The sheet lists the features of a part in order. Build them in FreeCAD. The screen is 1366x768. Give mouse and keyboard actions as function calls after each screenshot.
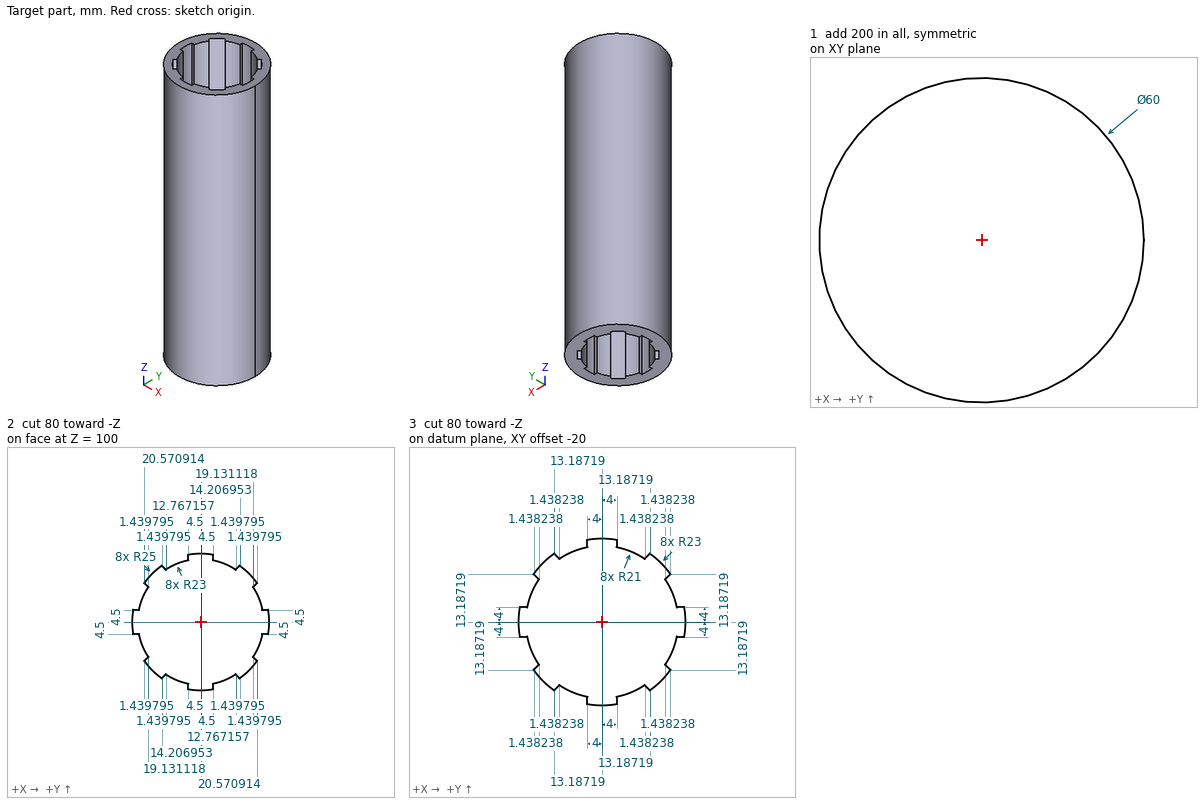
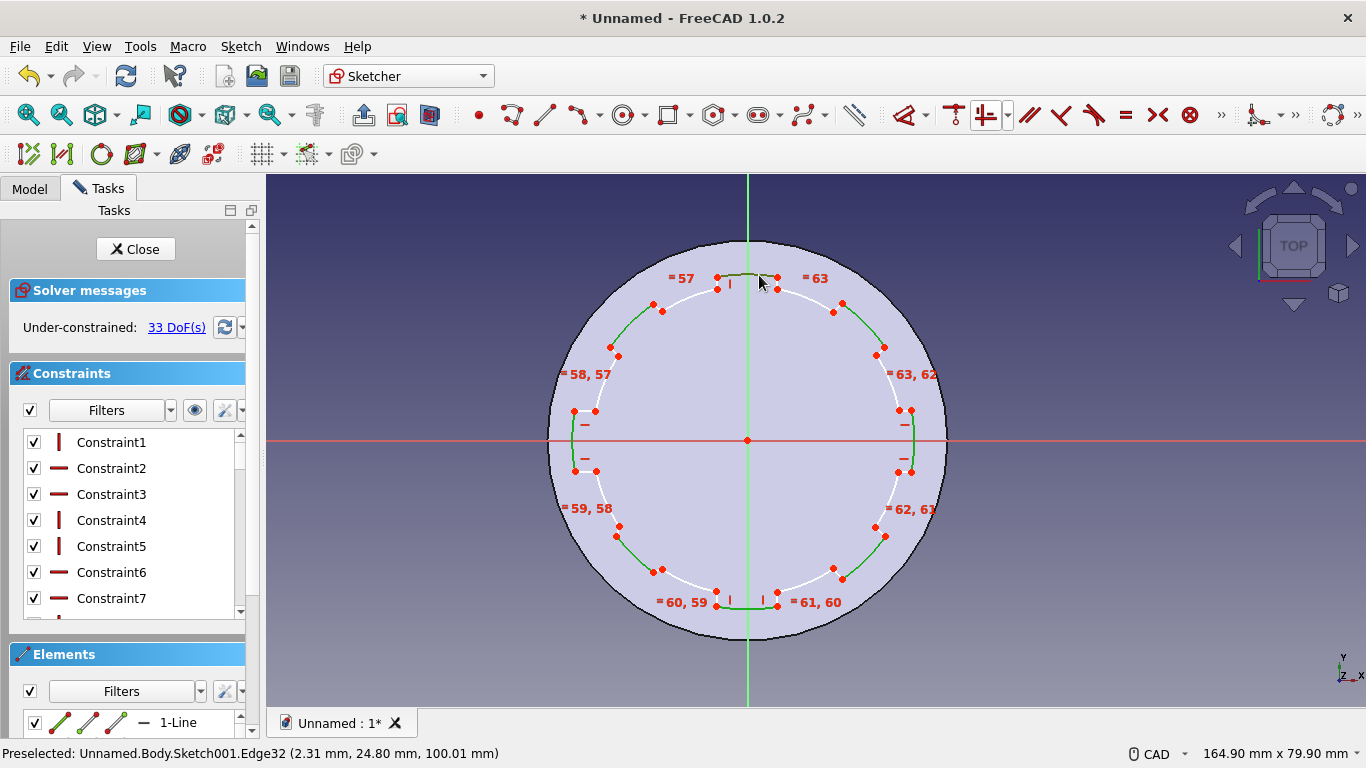
click(1126, 116)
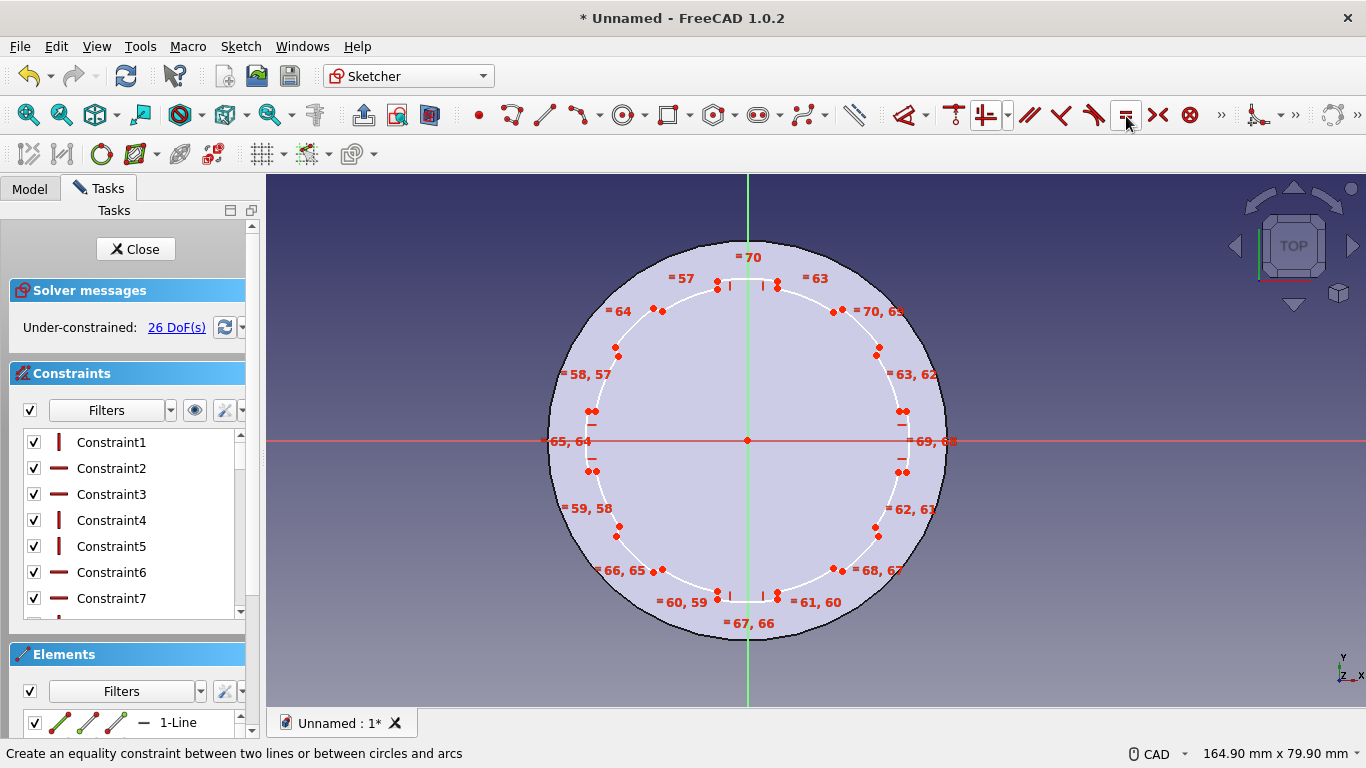
click(904, 116)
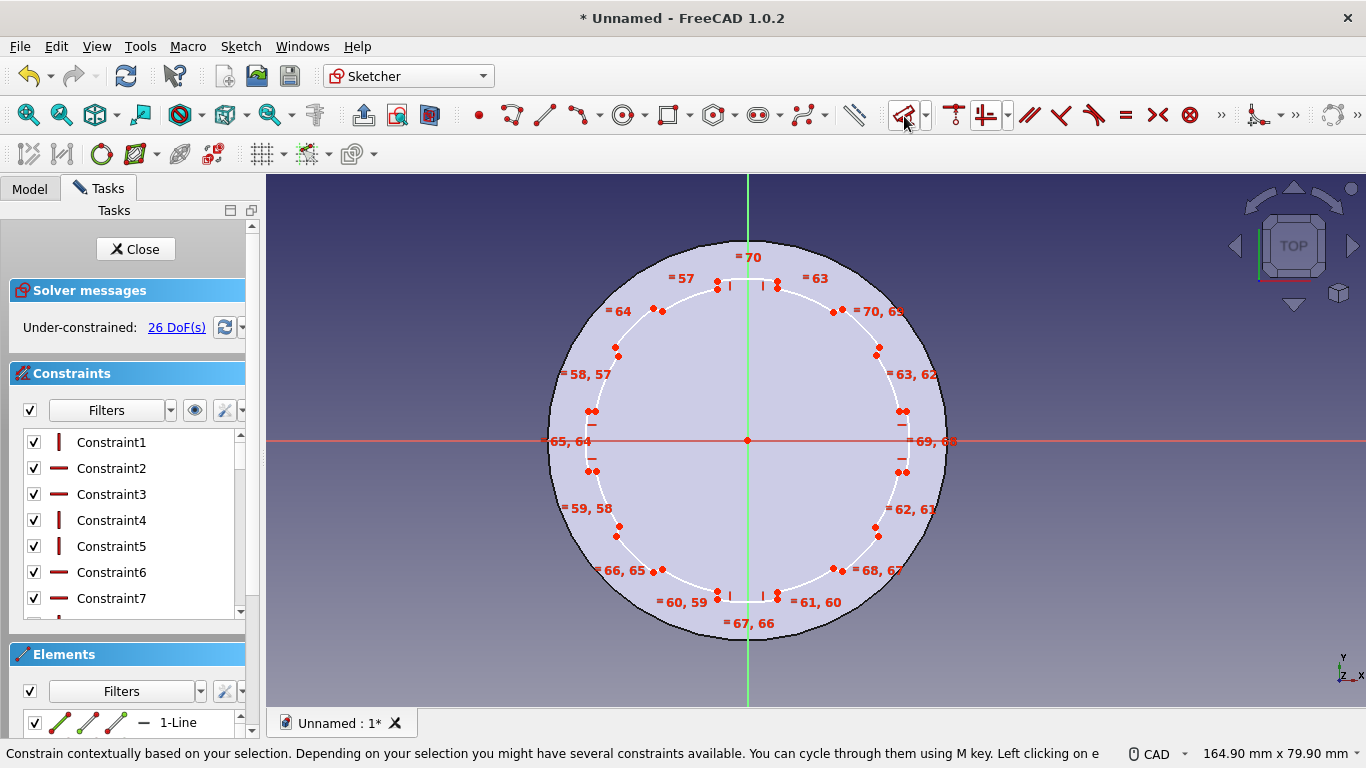
click(700, 294)
click(690, 264)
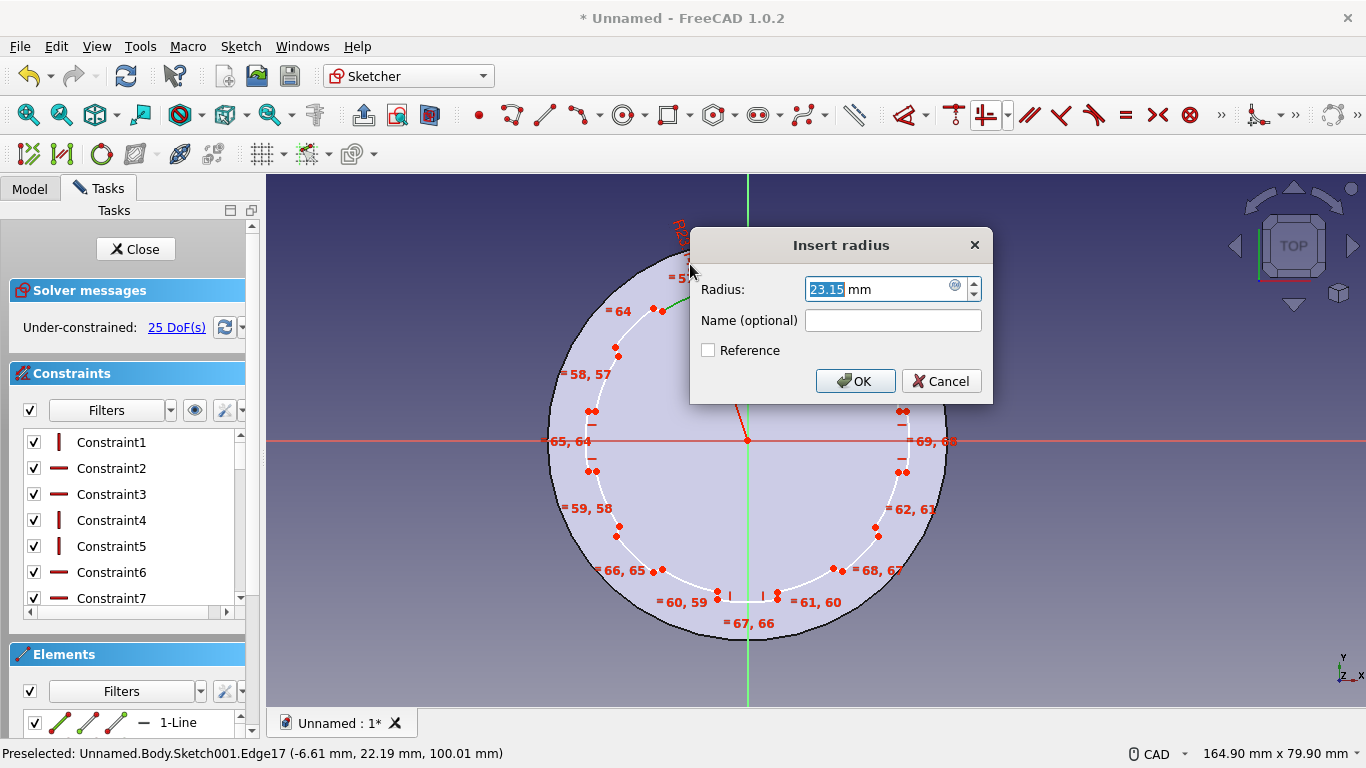
text(23)
key(Return)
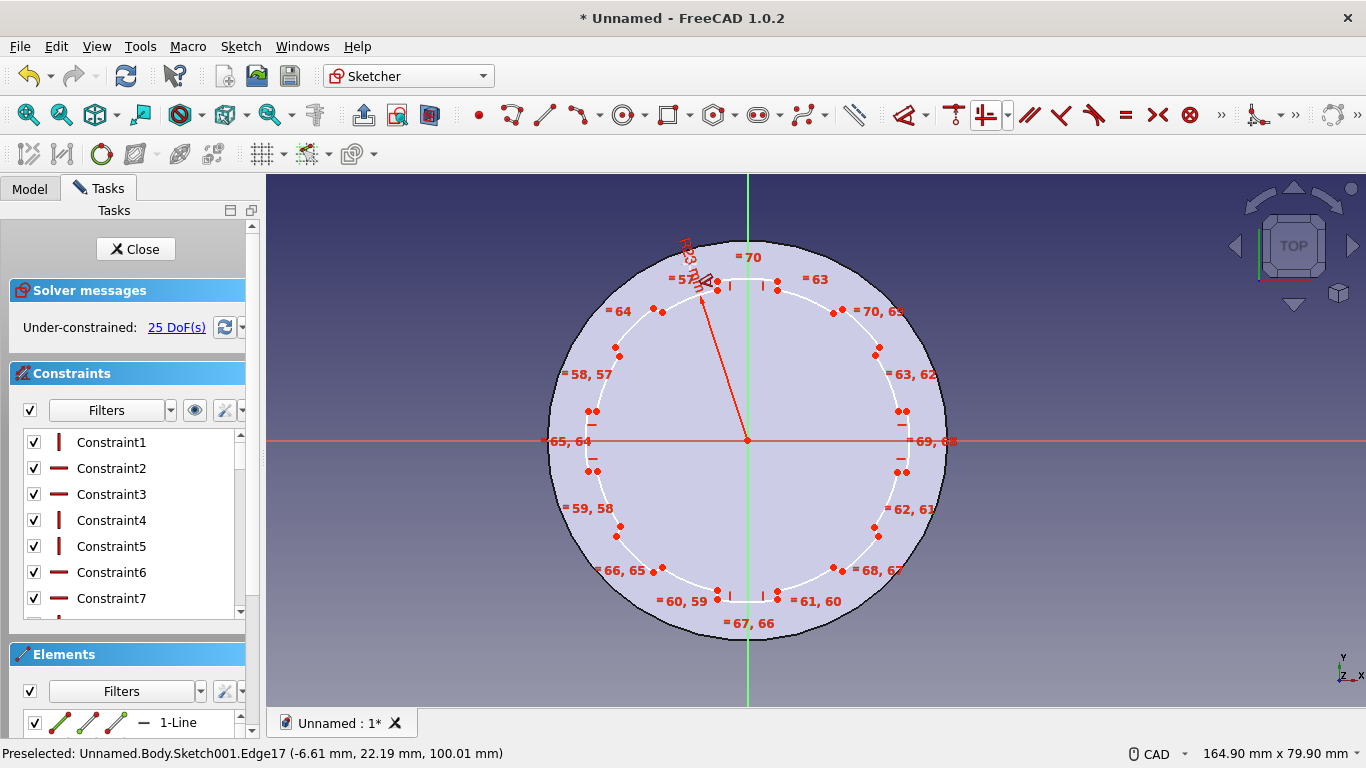
click(641, 319)
click(620, 295)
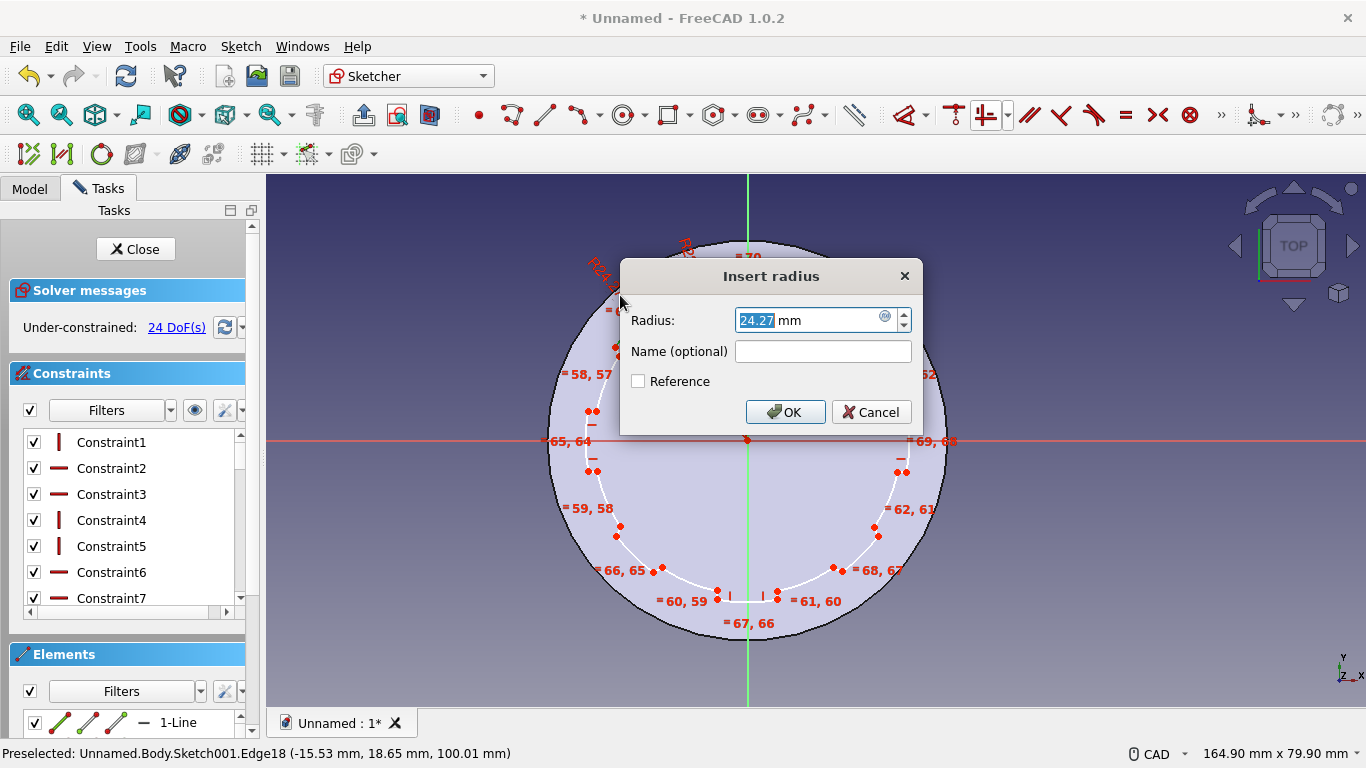
text(25)
key(Return)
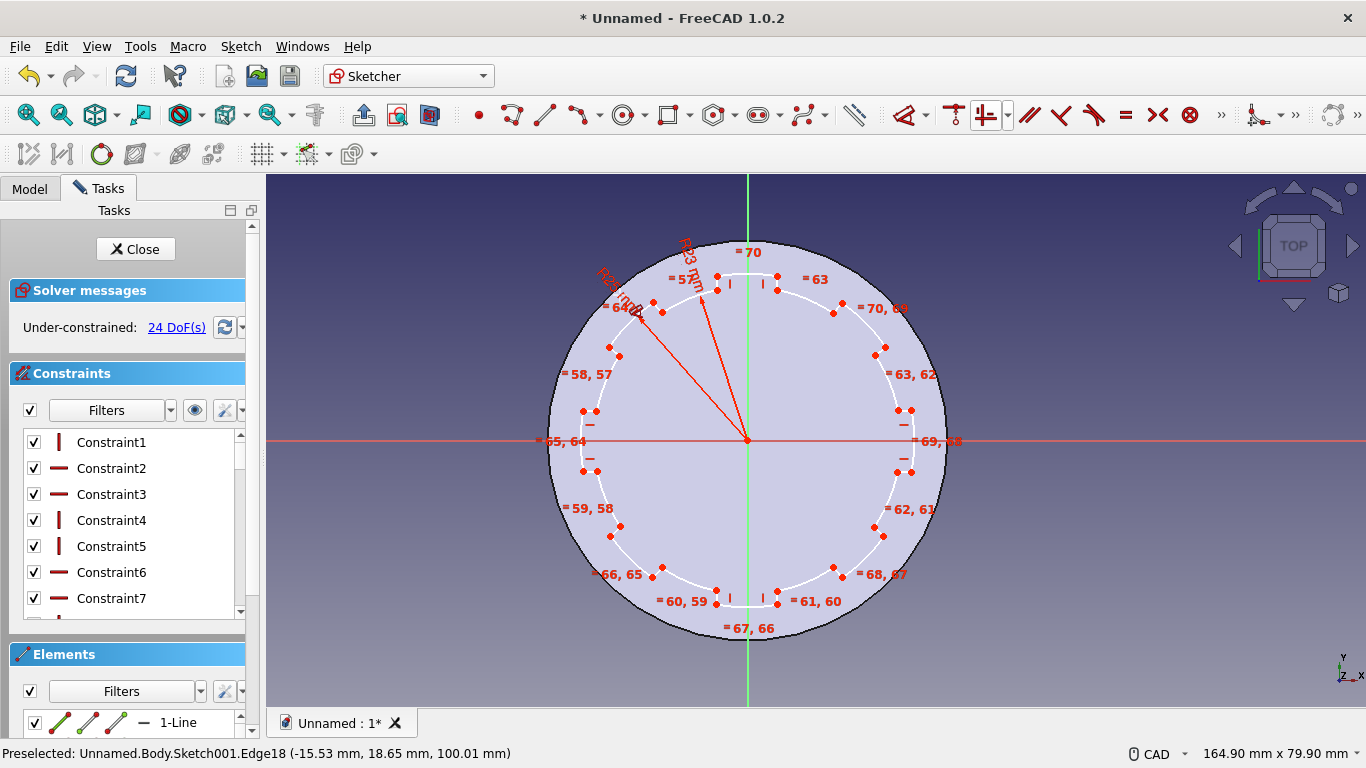
scroll(717, 277, up, 2)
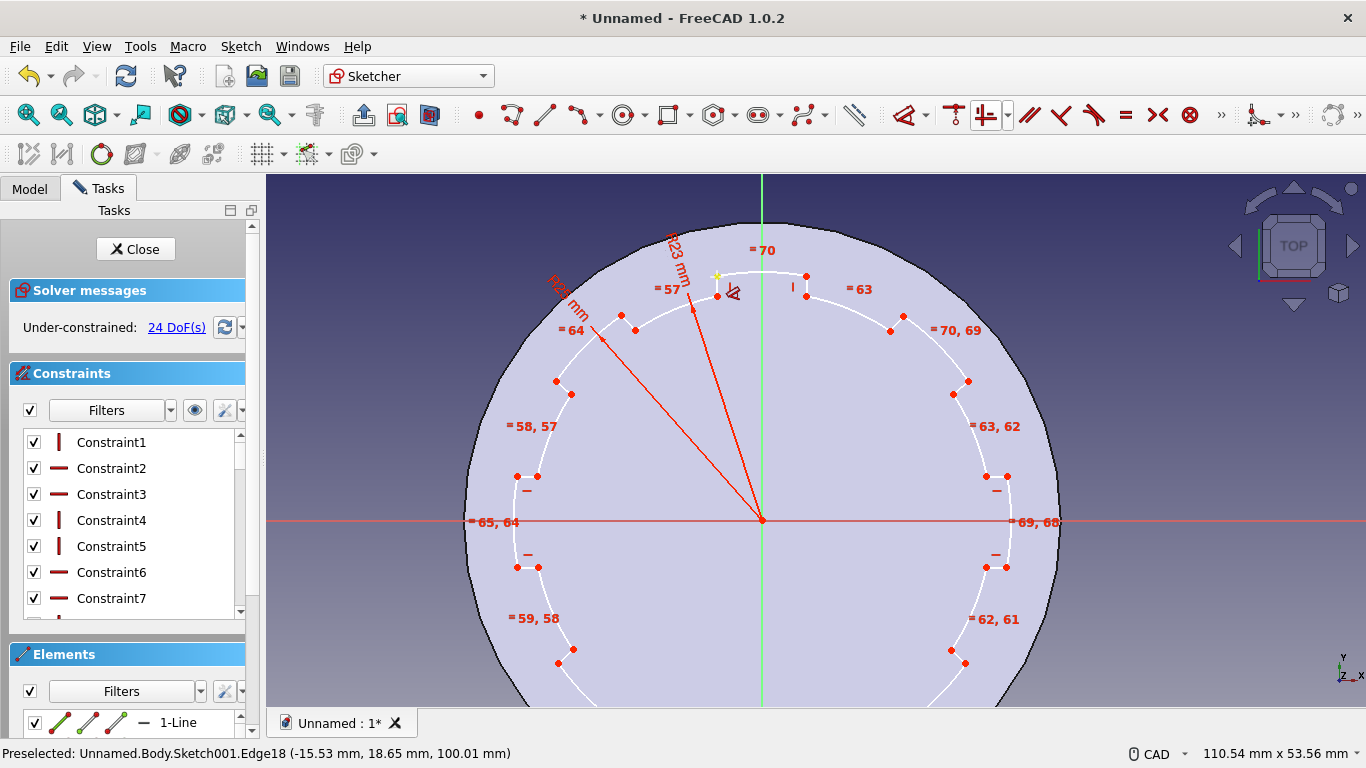
click(717, 276)
click(740, 555)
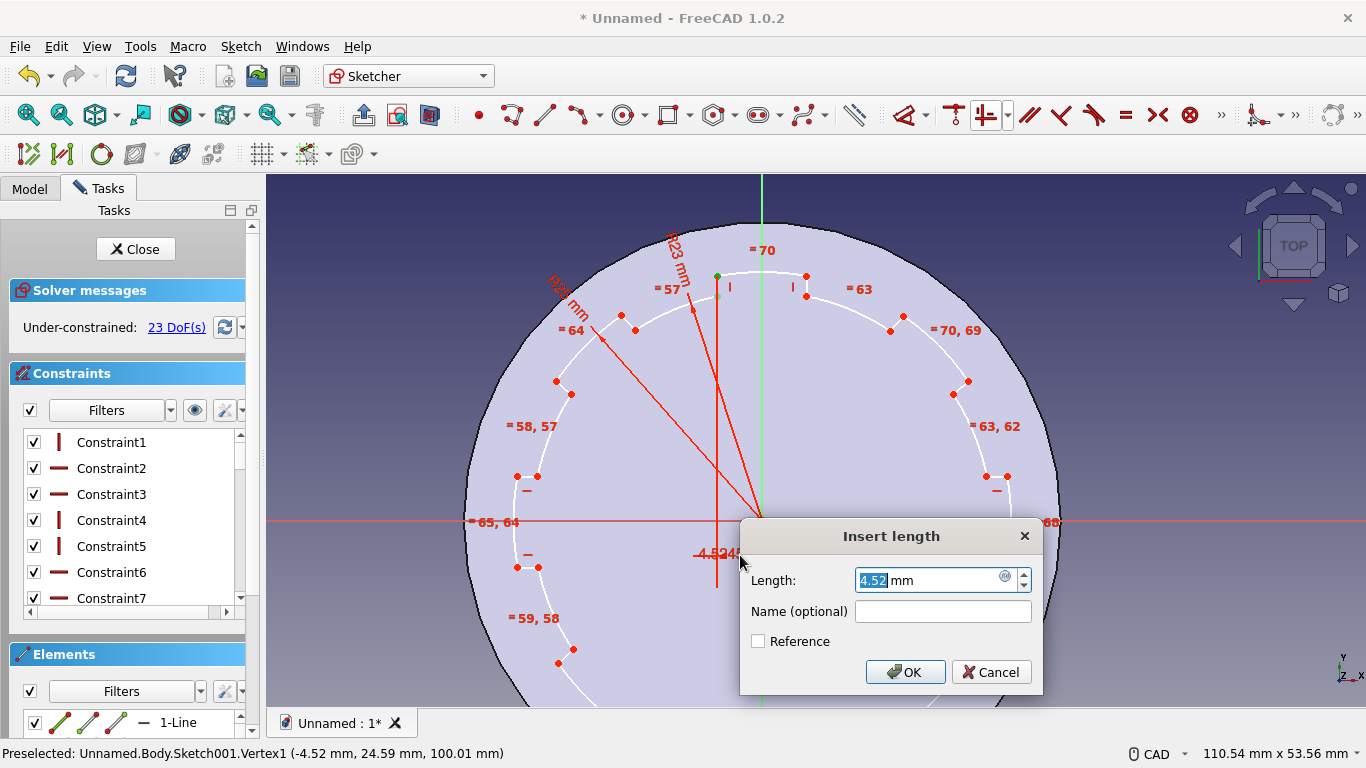
text(4.5)
key(Return)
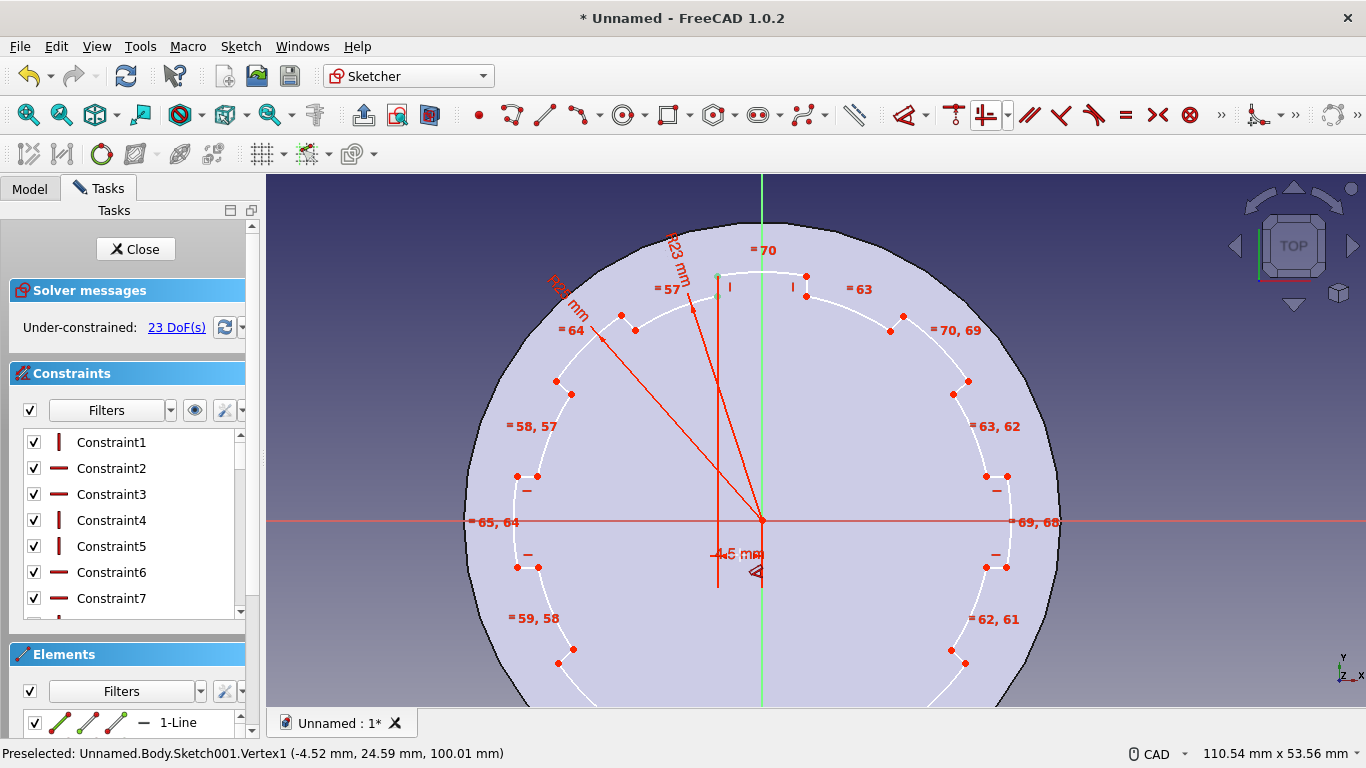
click(538, 477)
click(796, 499)